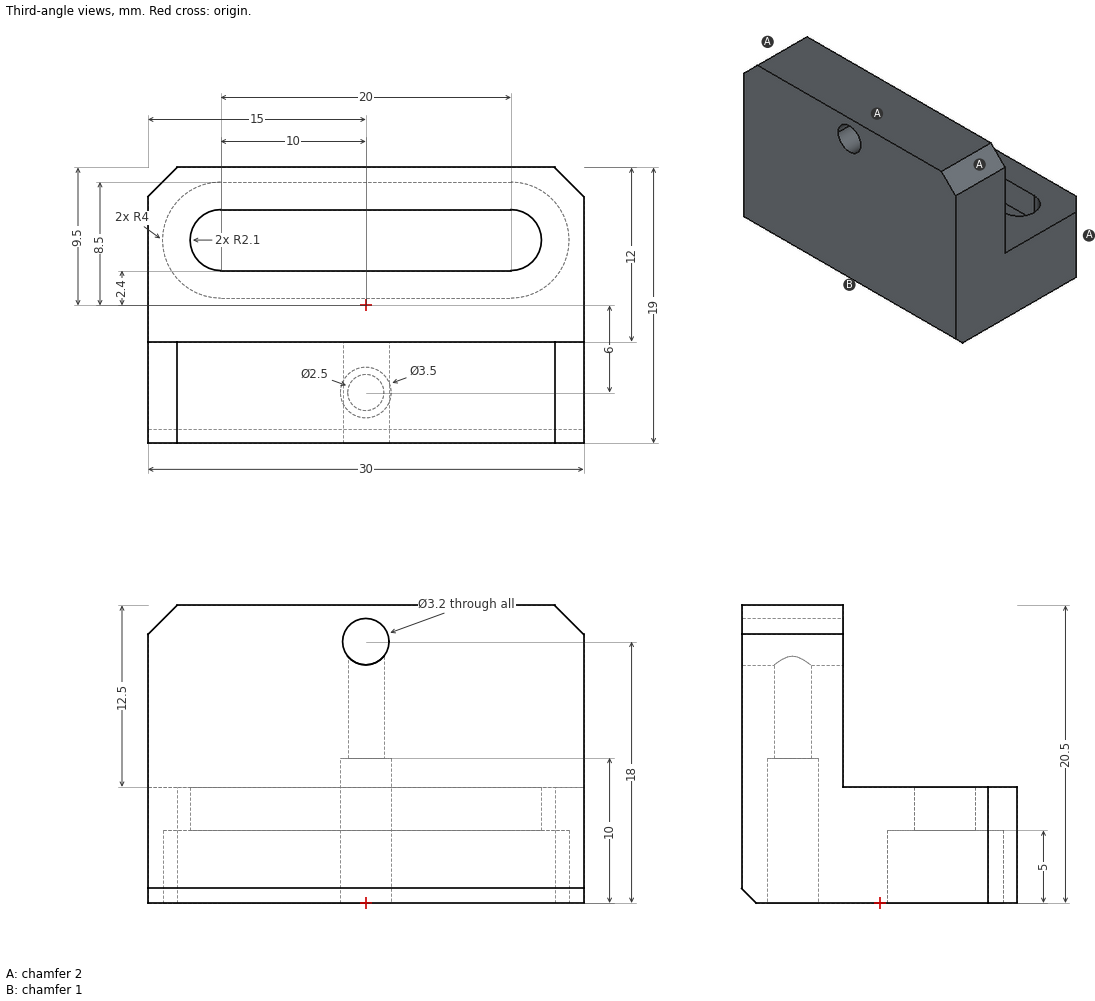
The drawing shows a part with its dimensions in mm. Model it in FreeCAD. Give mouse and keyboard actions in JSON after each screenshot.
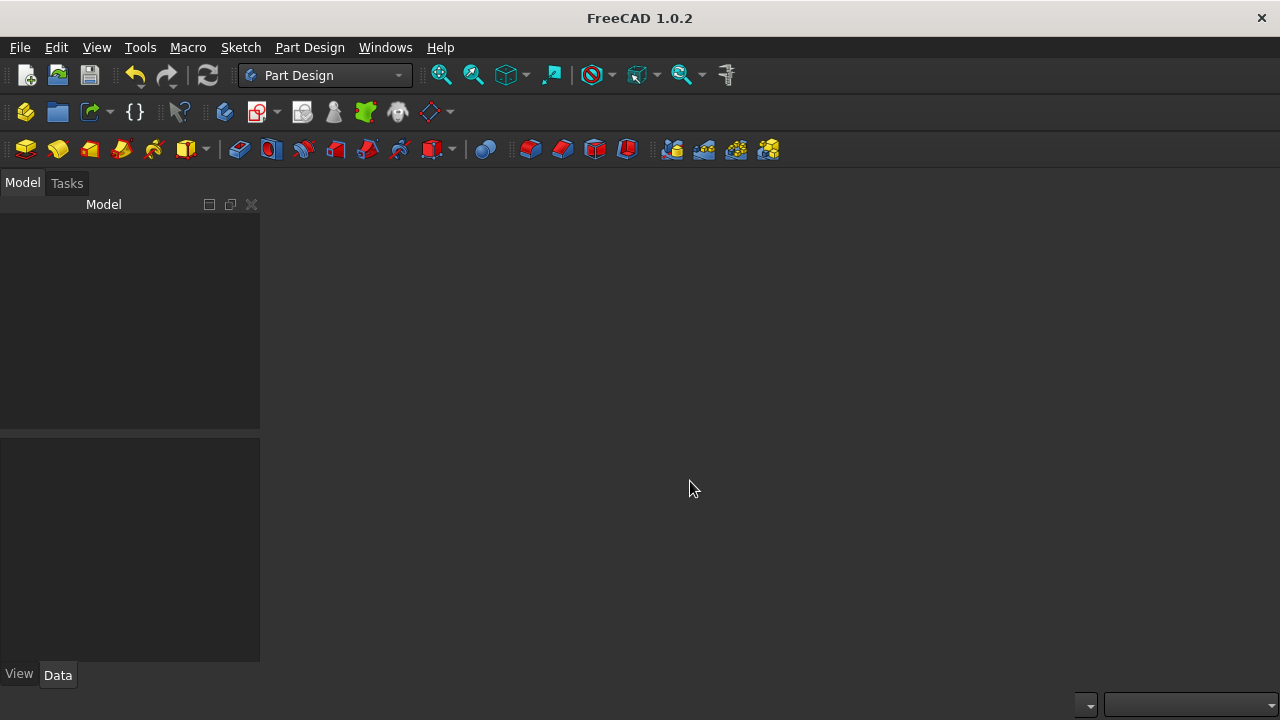
{"action": "left_click", "coordinate": [26, 76]}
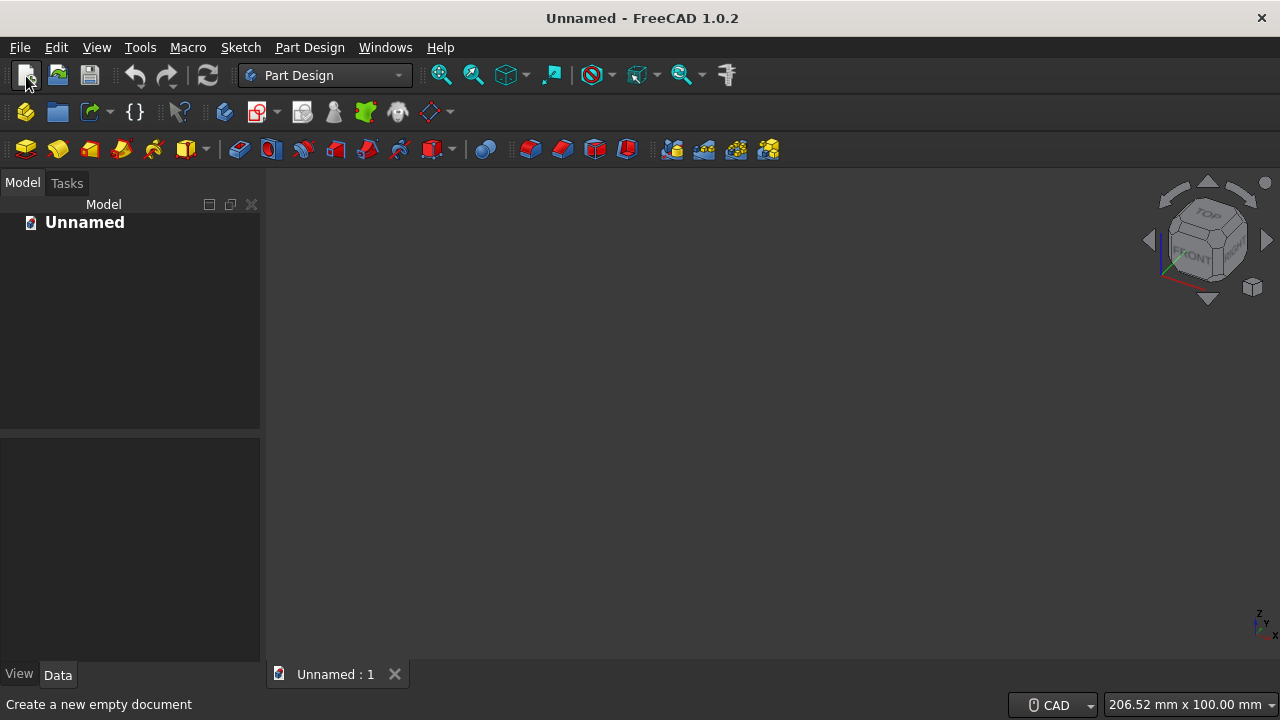
{"action": "left_click", "coordinate": [258, 112]}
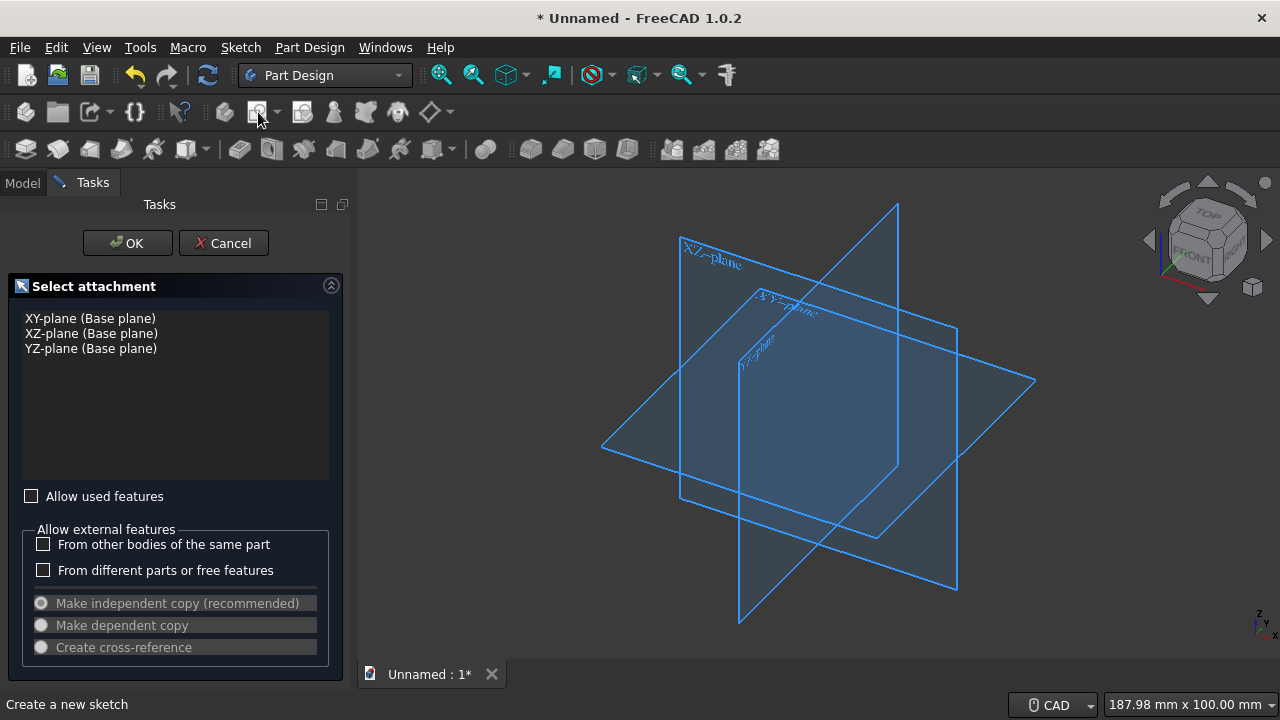
{"action": "left_click", "coordinate": [82, 318]}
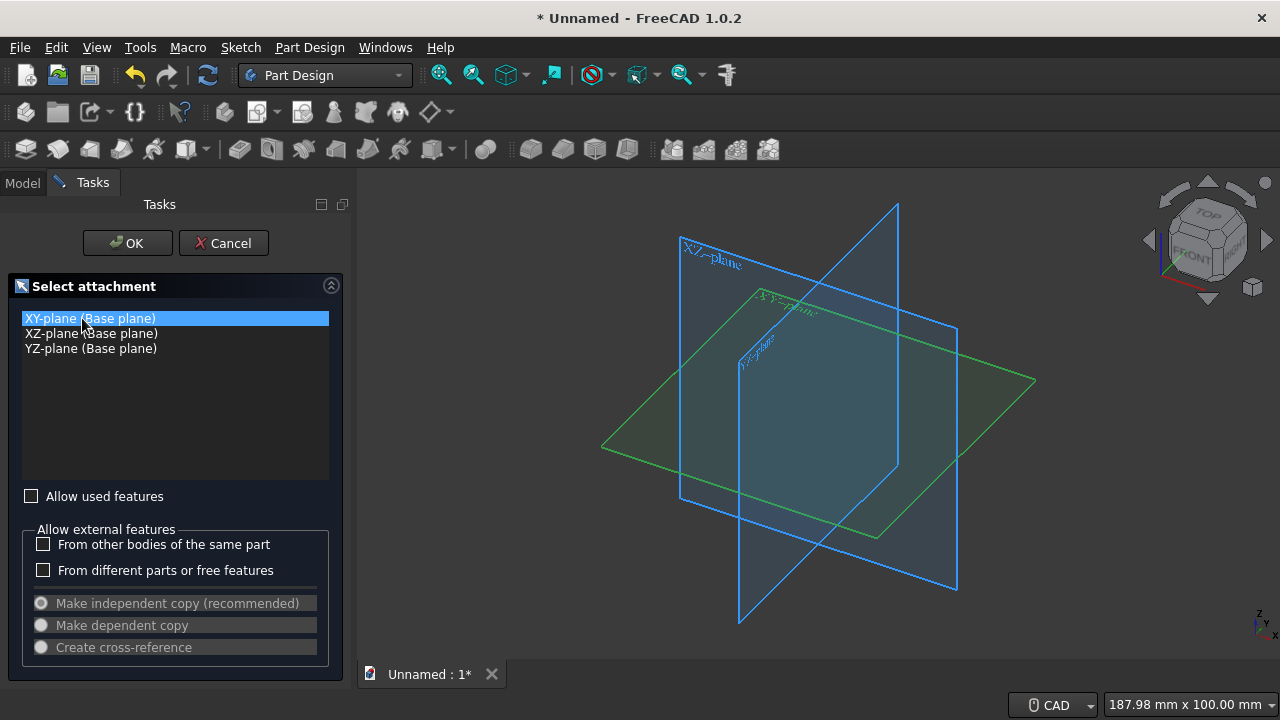
{"action": "left_click", "coordinate": [128, 243]}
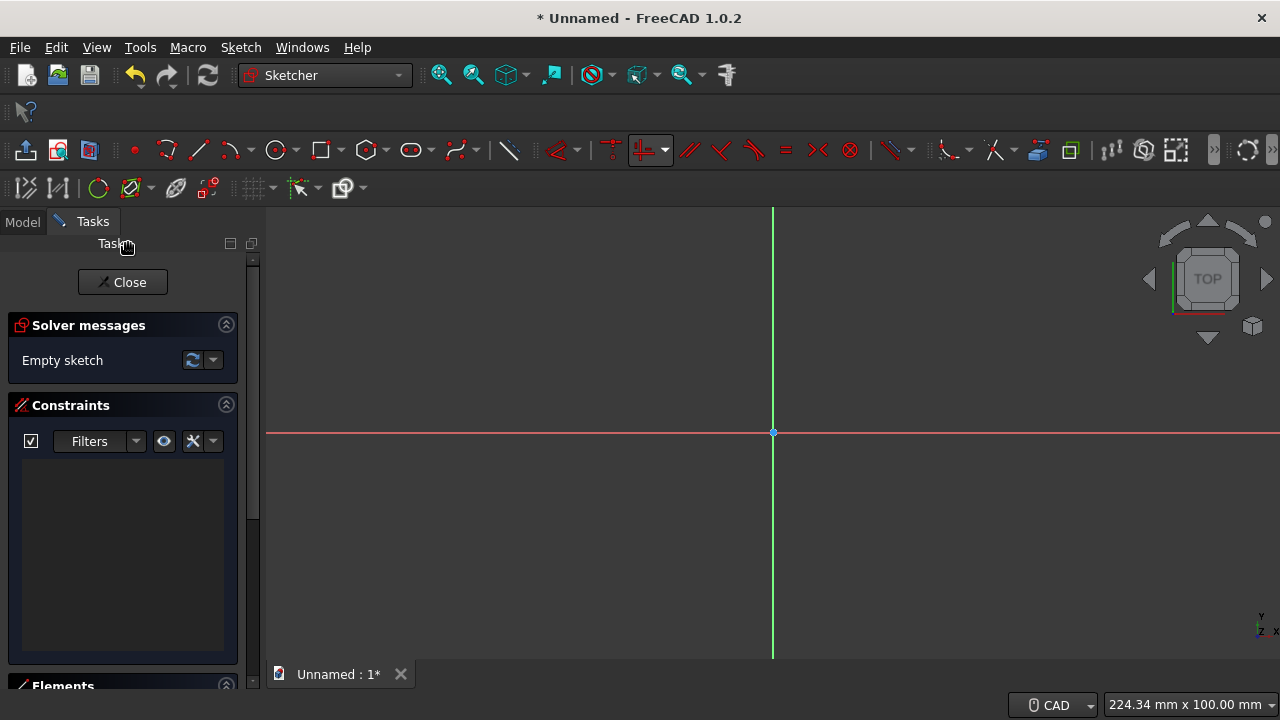
{"action": "scroll", "coordinate": [803, 433], "scroll_direction": "up", "scroll_amount": 6}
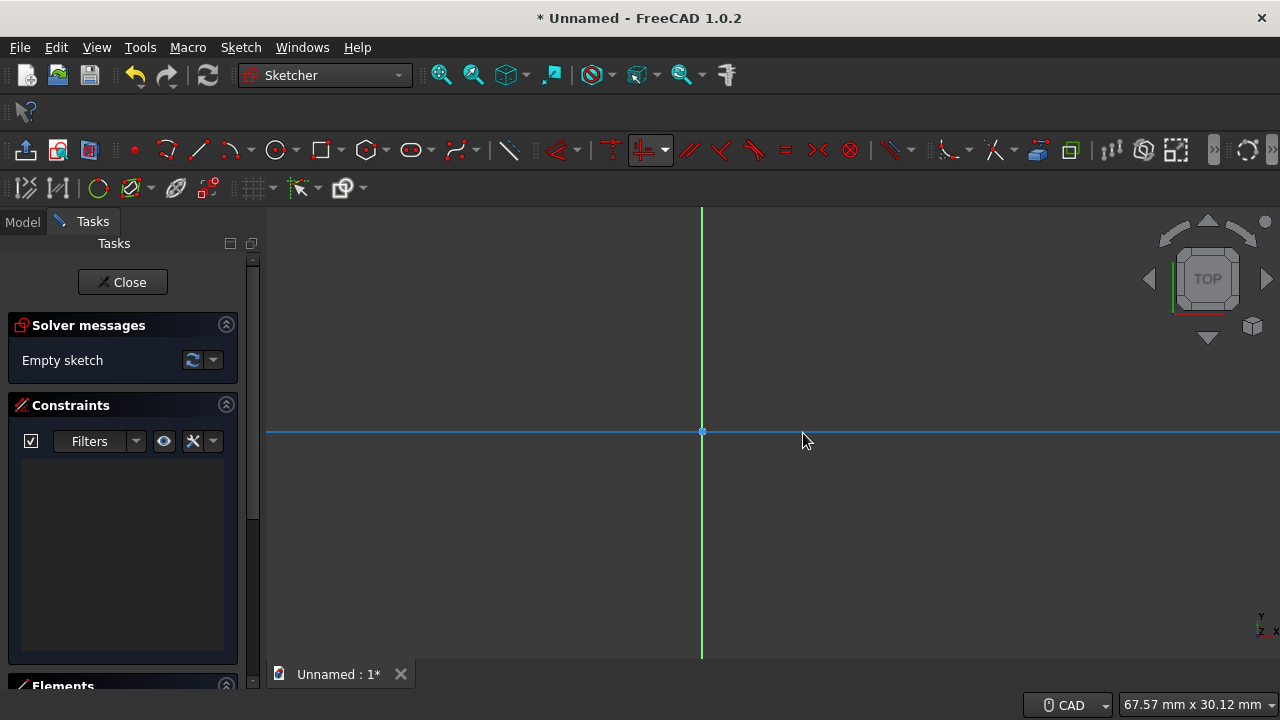
{"action": "left_click", "coordinate": [344, 150]}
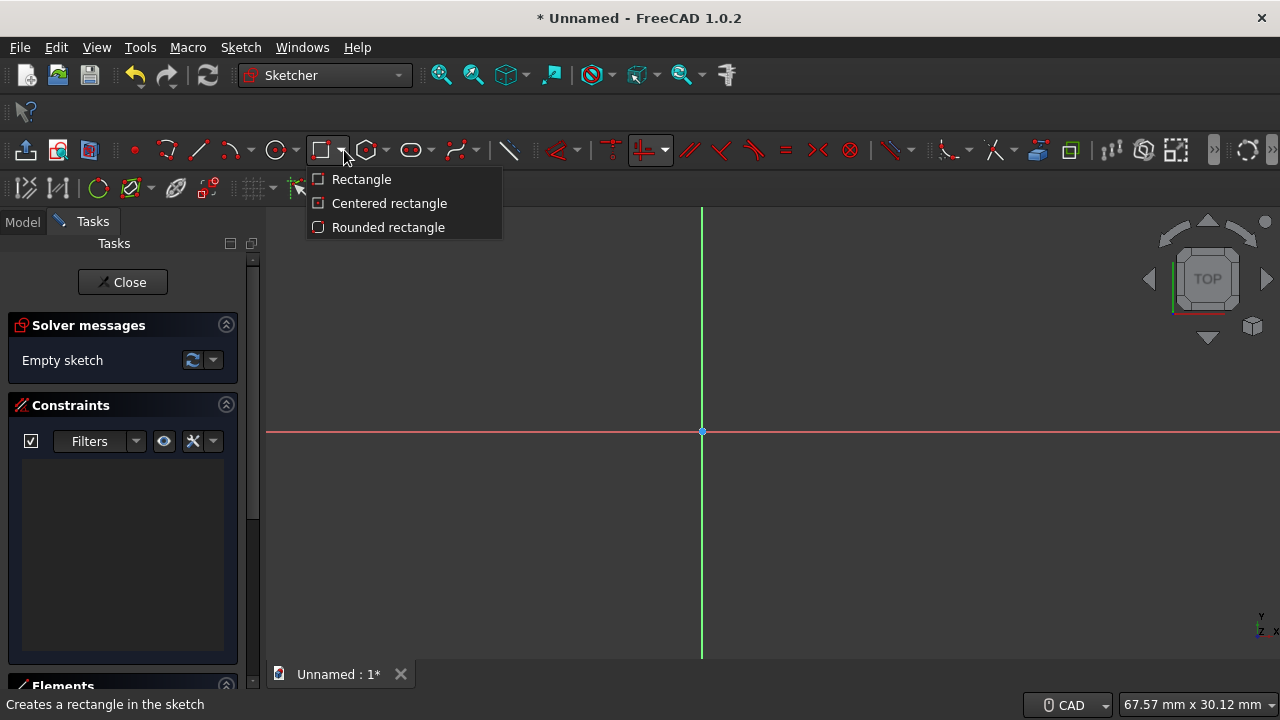
{"action": "left_click", "coordinate": [404, 203]}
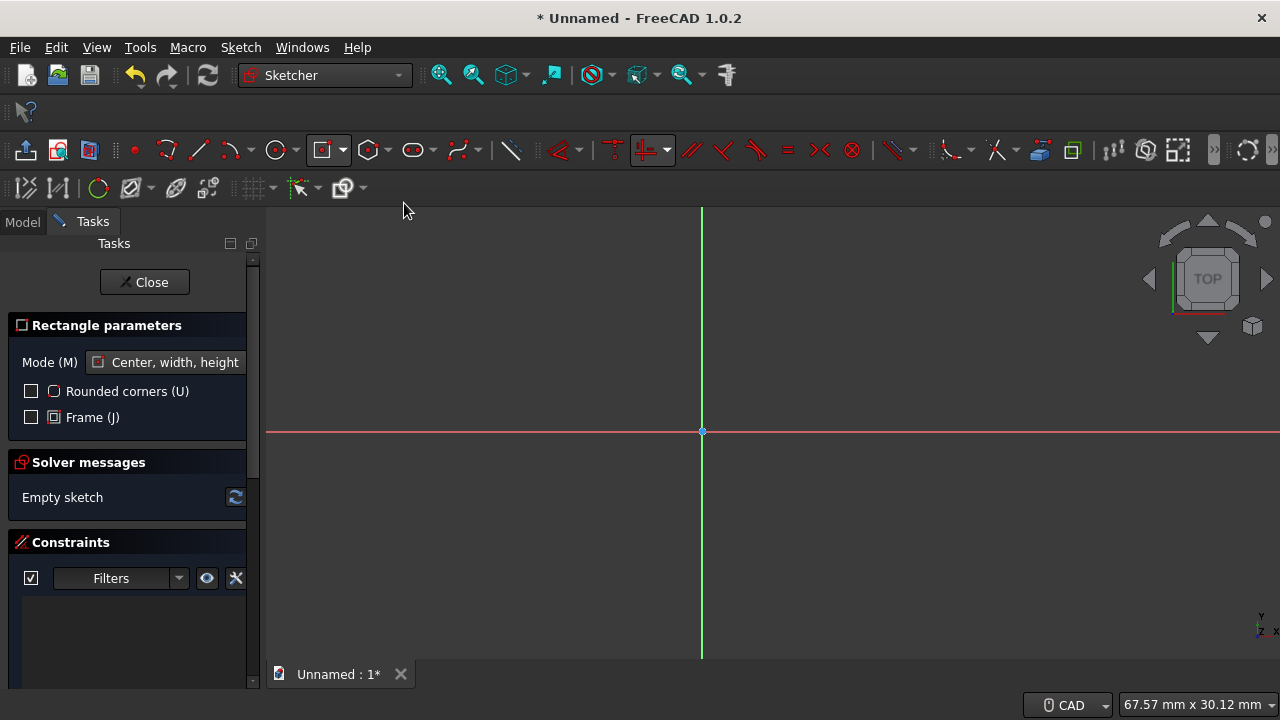
{"action": "left_click", "coordinate": [702, 432]}
{"action": "mouse_move", "coordinate": [927, 289]}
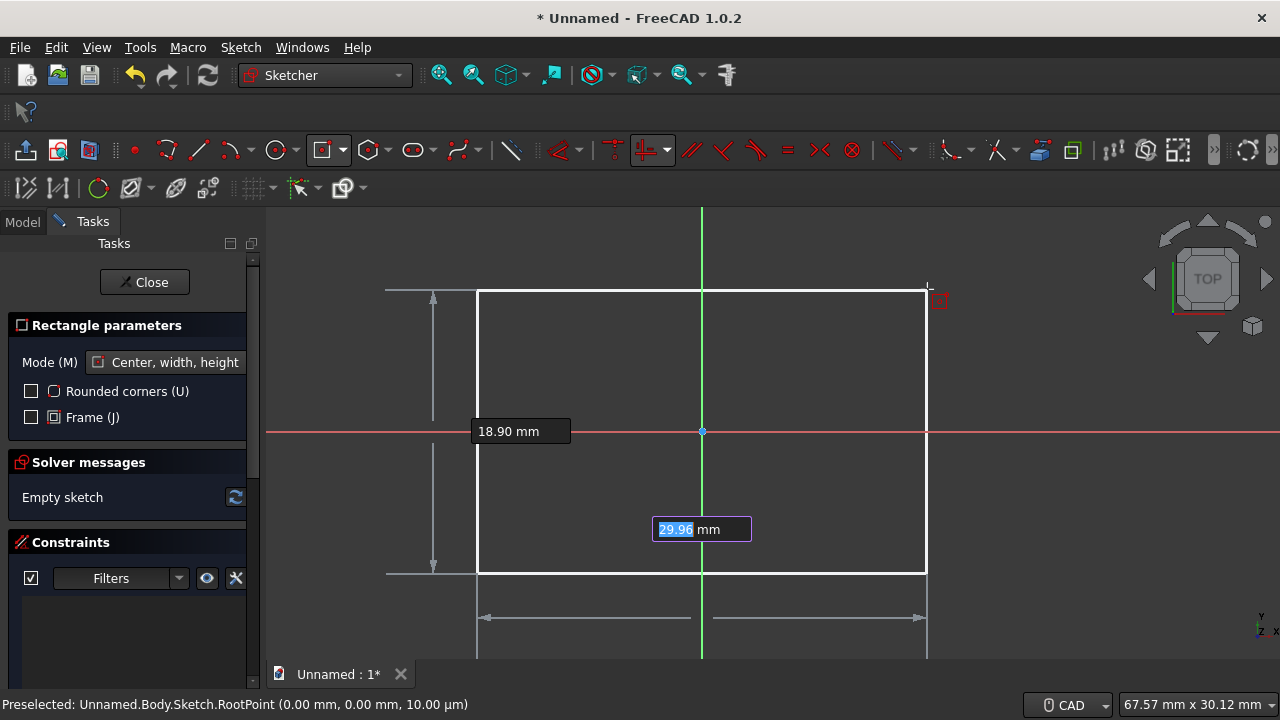
{"action": "type", "text": "30"}
{"action": "key", "text": "Tab"}
{"action": "type", "text": "19"}
{"action": "key", "text": "Return"}
{"action": "key", "text": "Escape"}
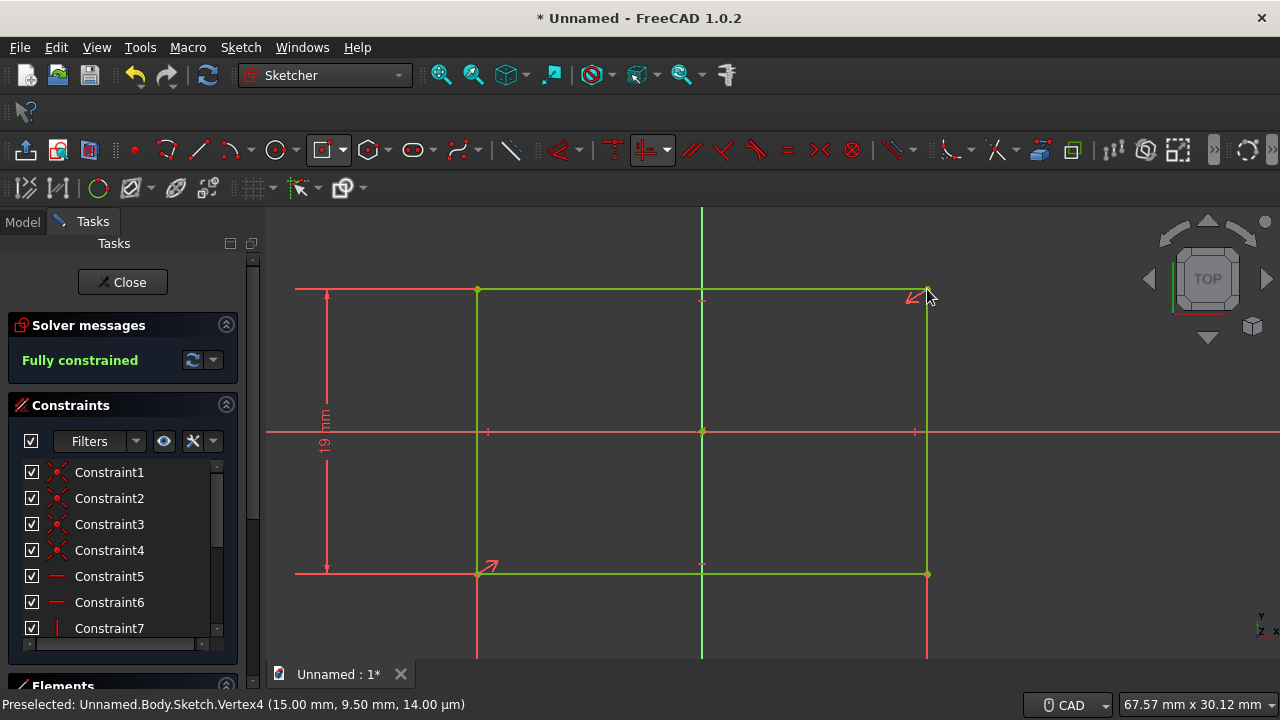
{"action": "left_click", "coordinate": [123, 282]}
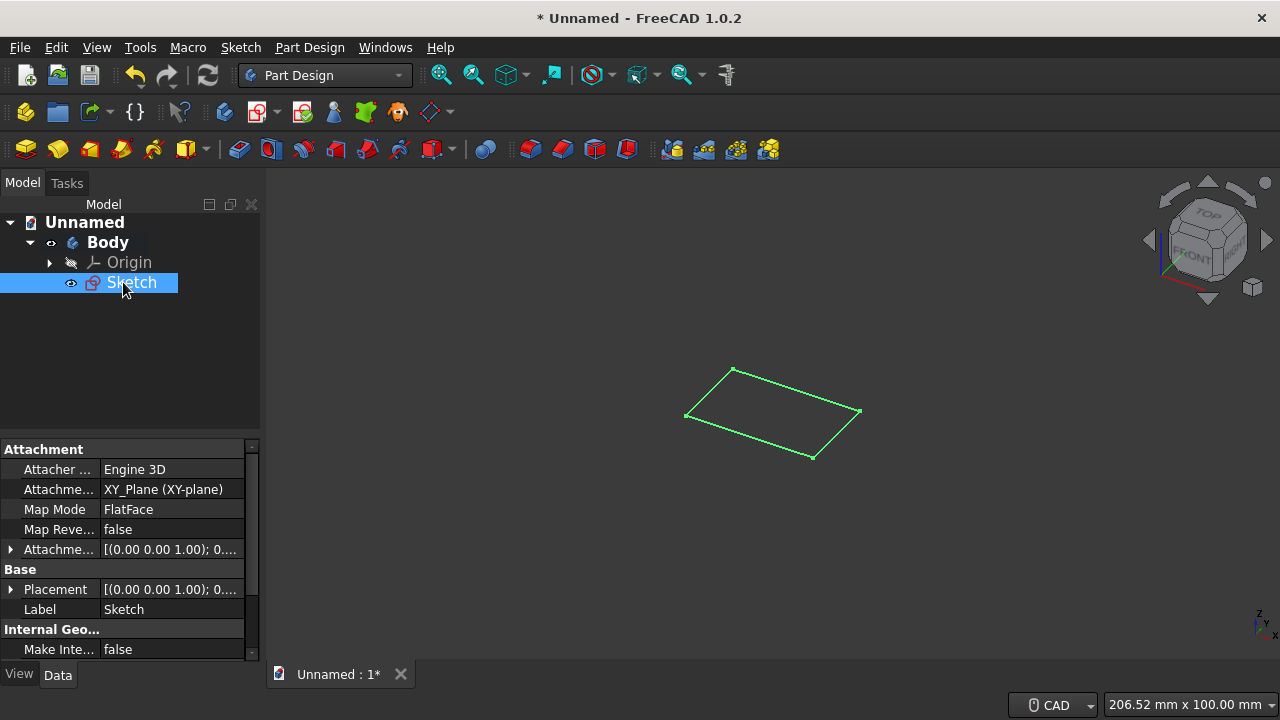
{"action": "left_click", "coordinate": [26, 150]}